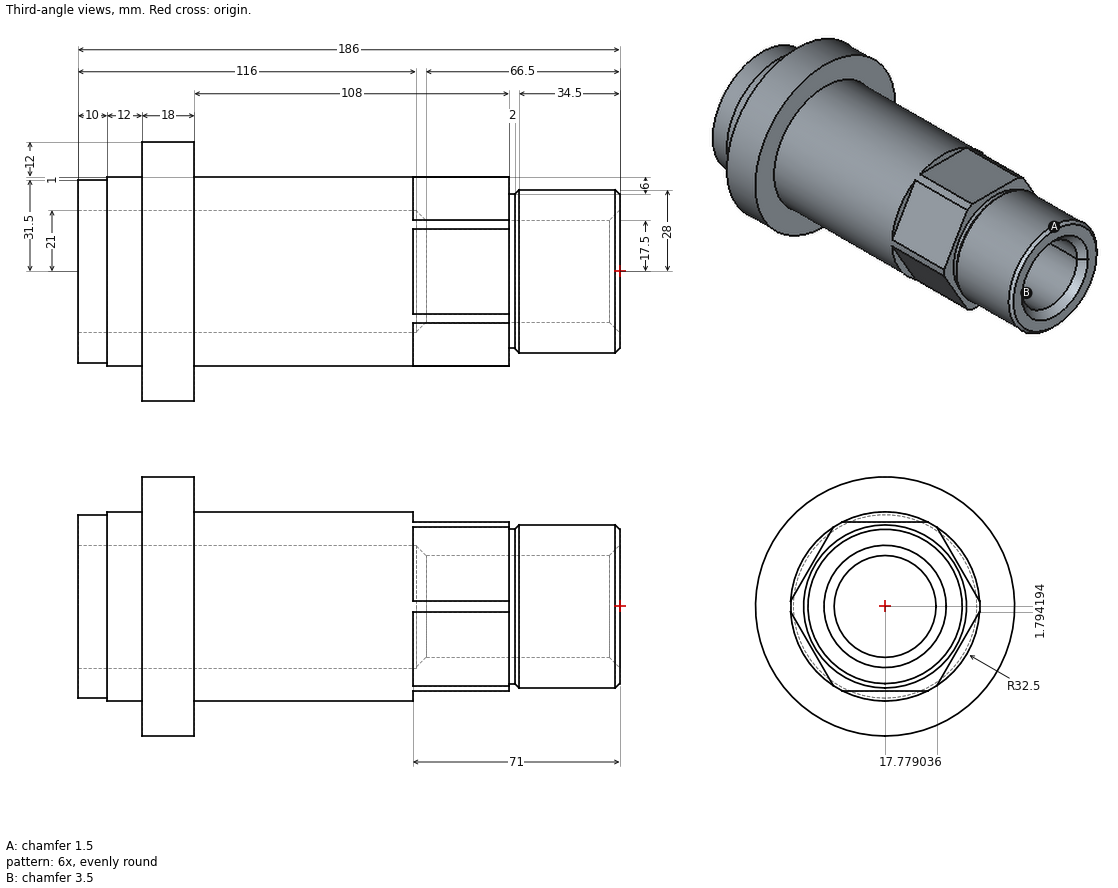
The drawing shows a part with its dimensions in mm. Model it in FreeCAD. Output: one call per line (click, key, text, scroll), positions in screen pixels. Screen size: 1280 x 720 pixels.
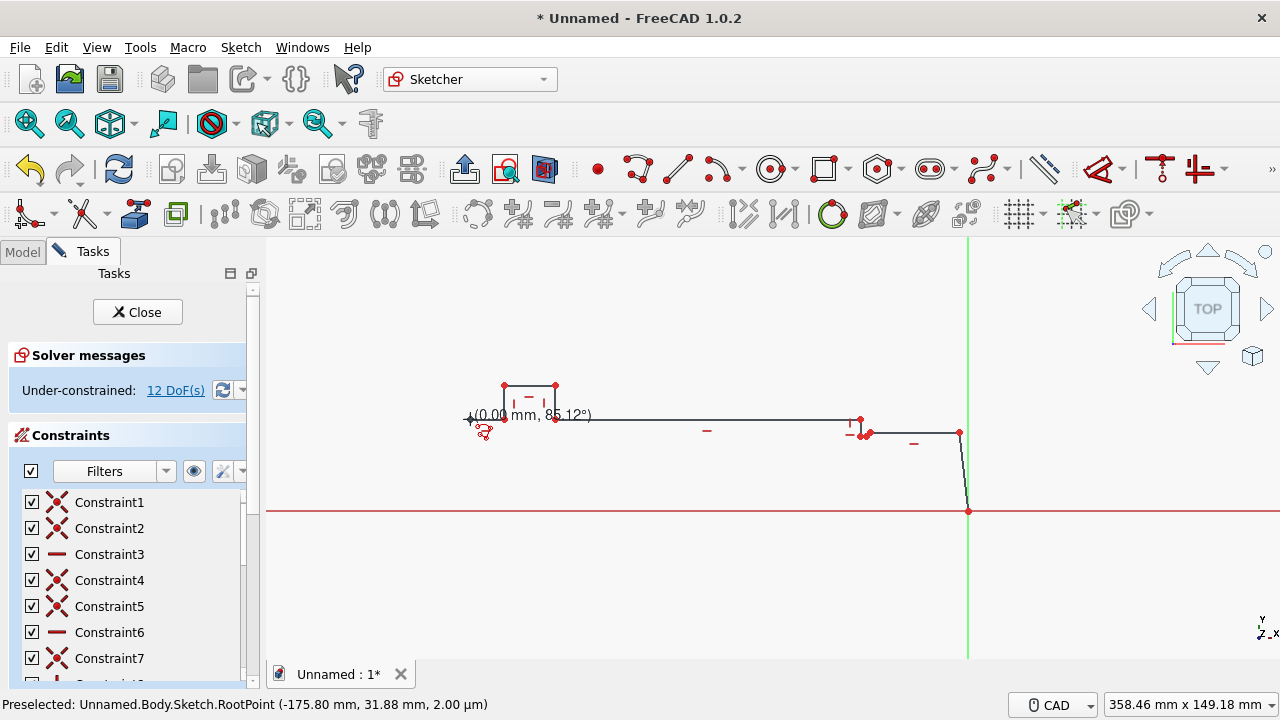
scroll(470, 422, up, 9)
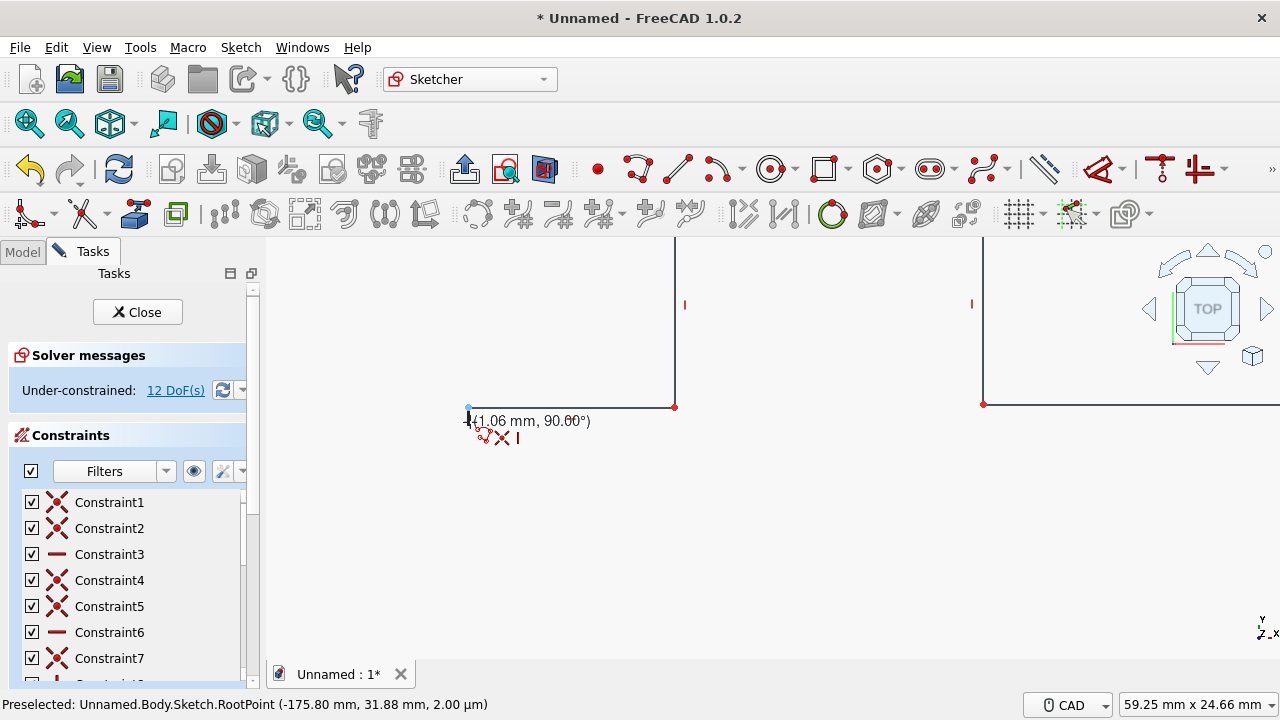
click(469, 420)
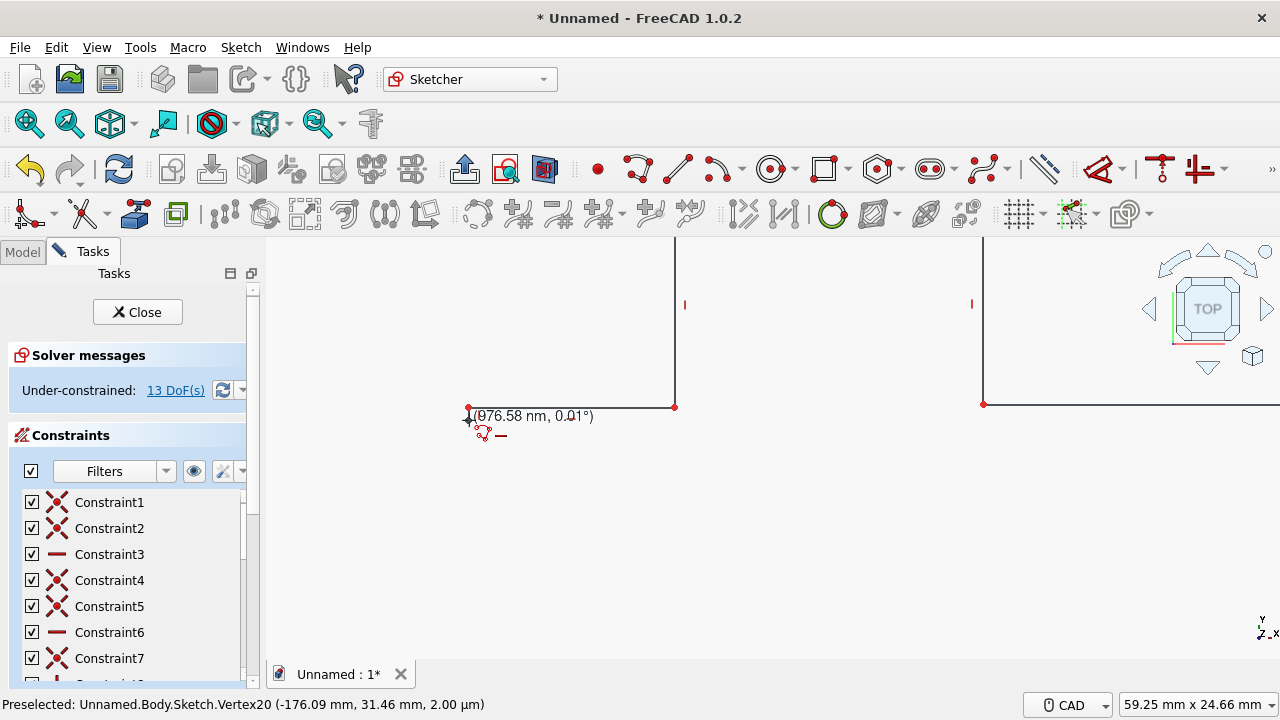
scroll(469, 422, down, 9)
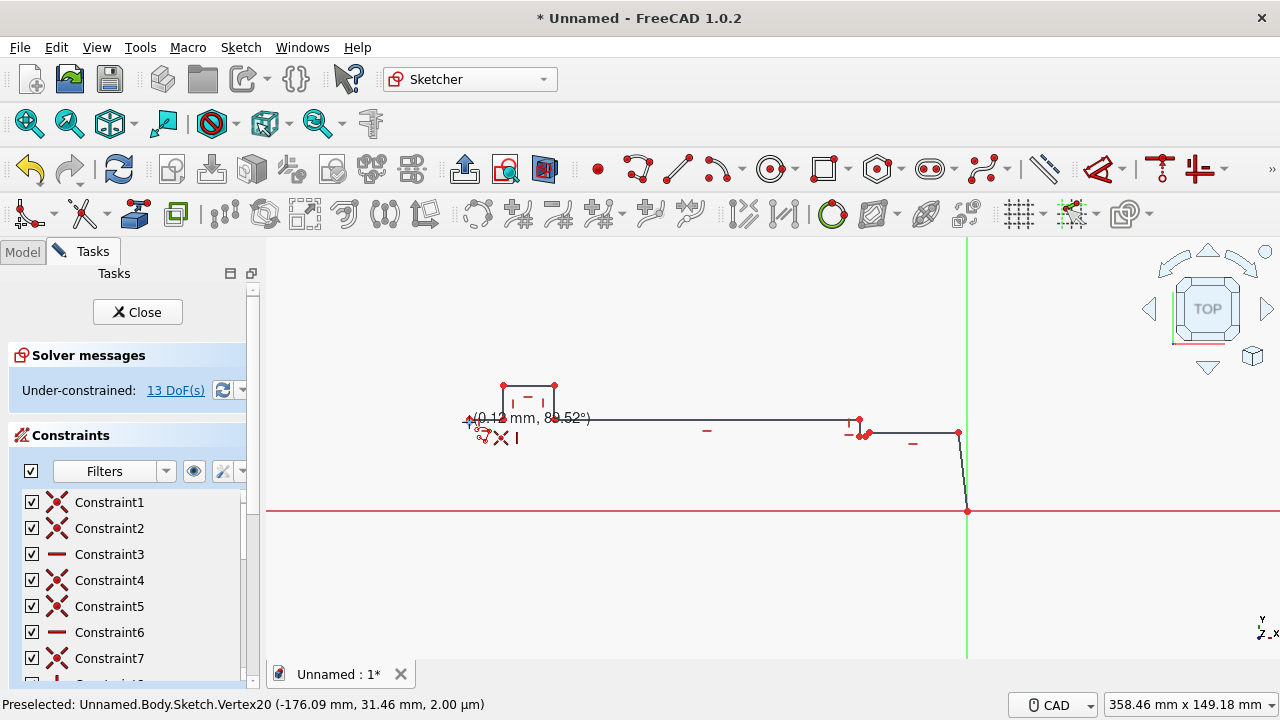
click(441, 422)
click(441, 502)
click(967, 511)
key(Escape)
key(Escape)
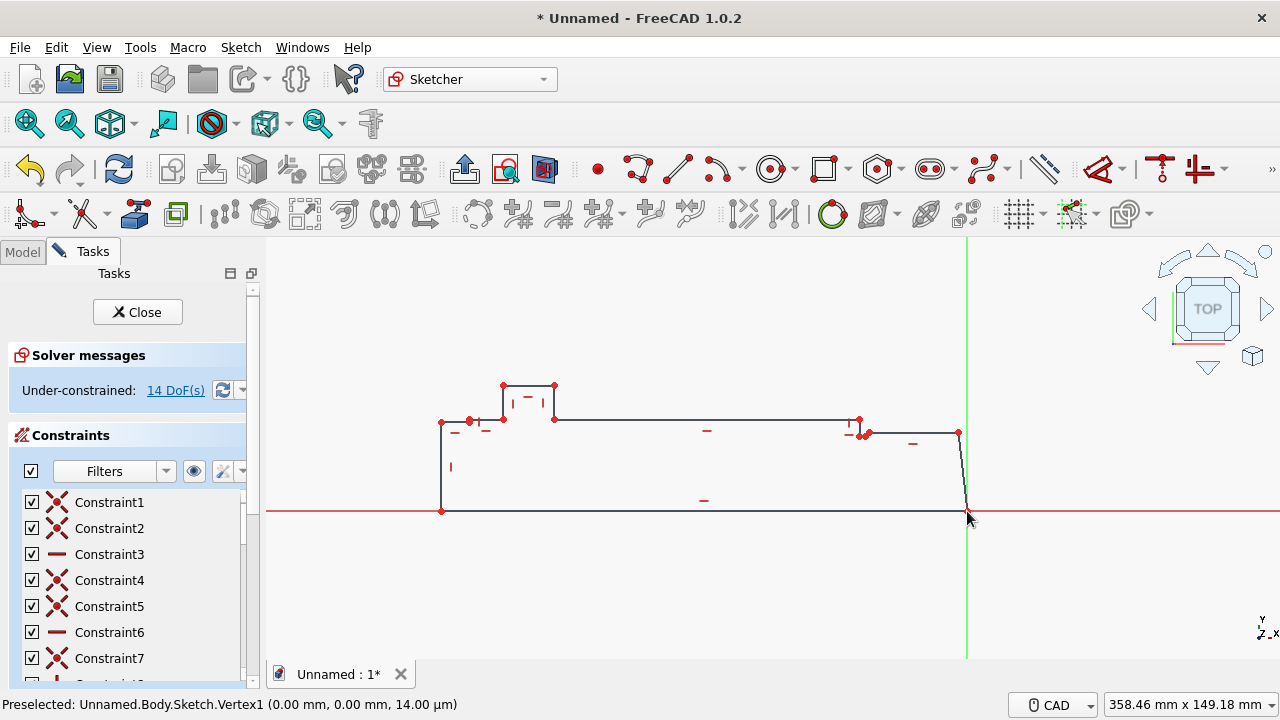
click(965, 488)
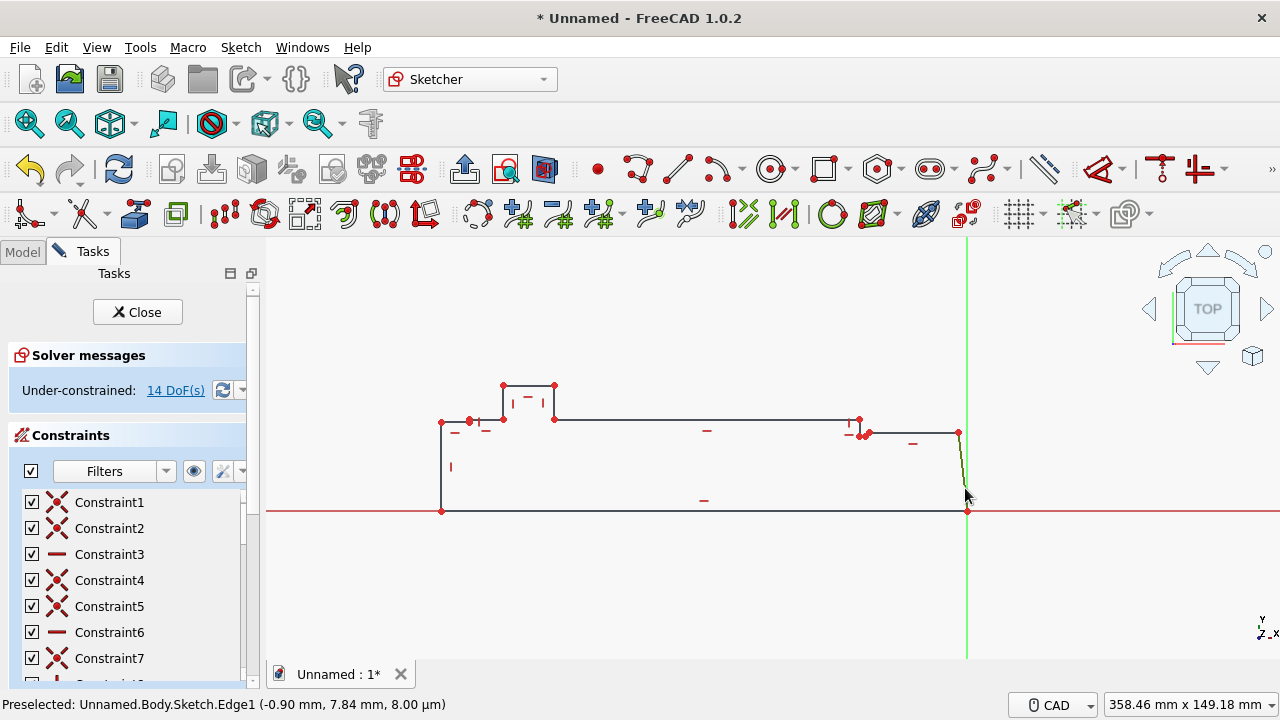
click(1226, 170)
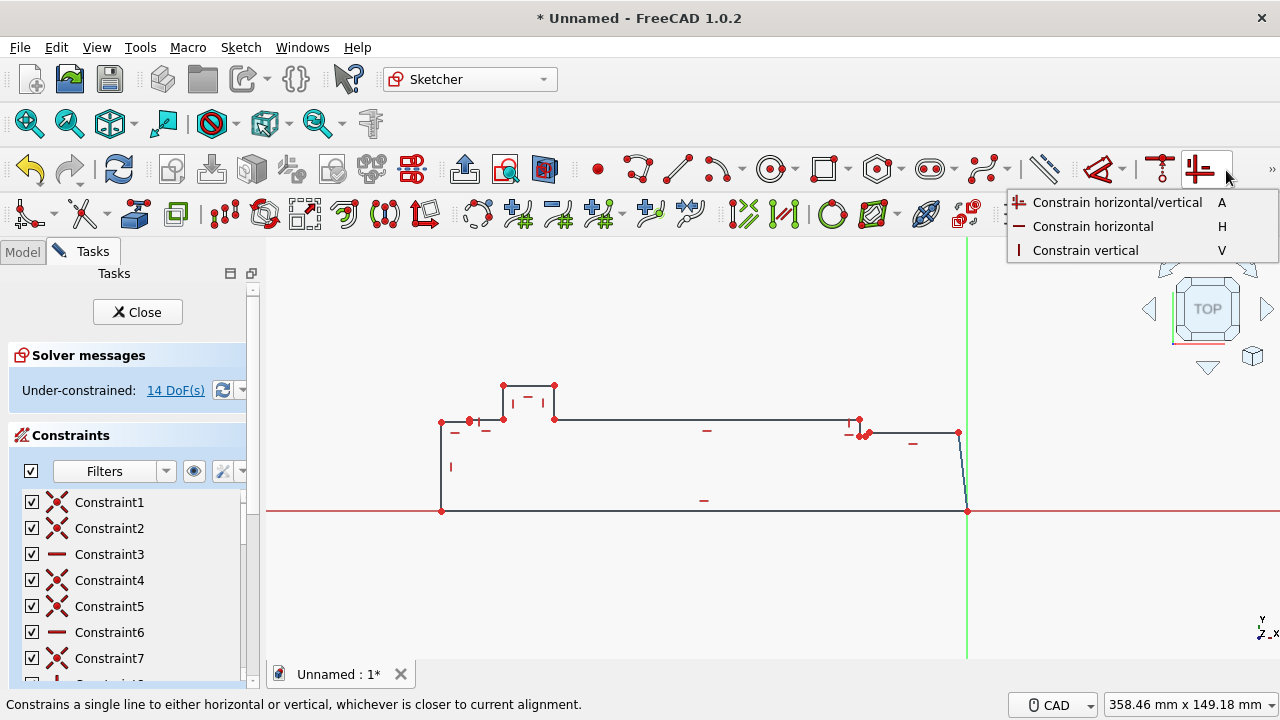
click(1143, 250)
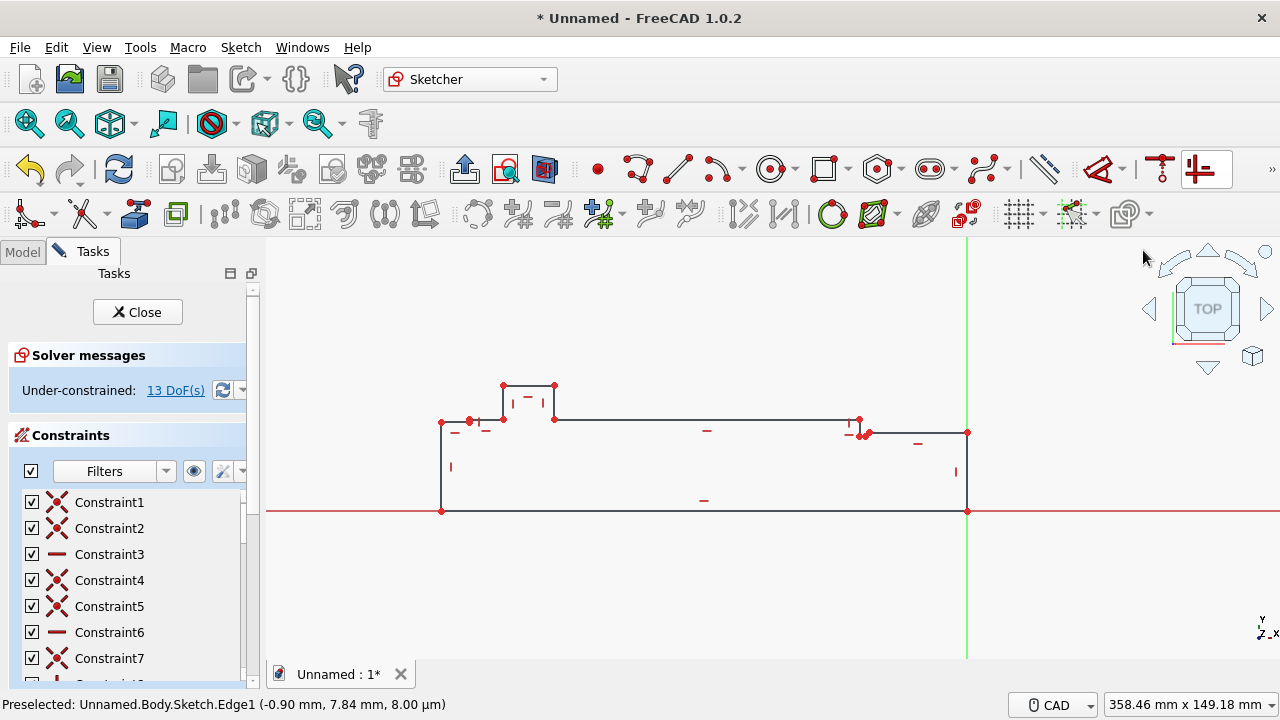
click(1098, 170)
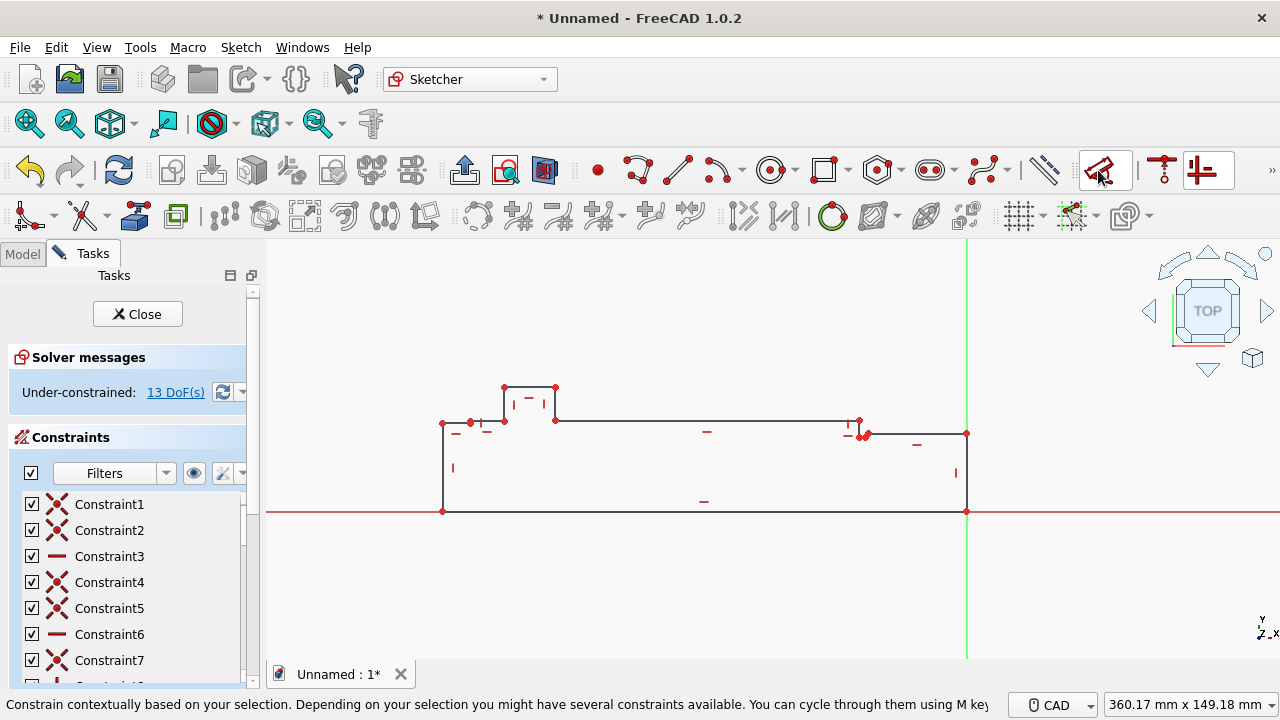
scroll(862, 438, up, 10)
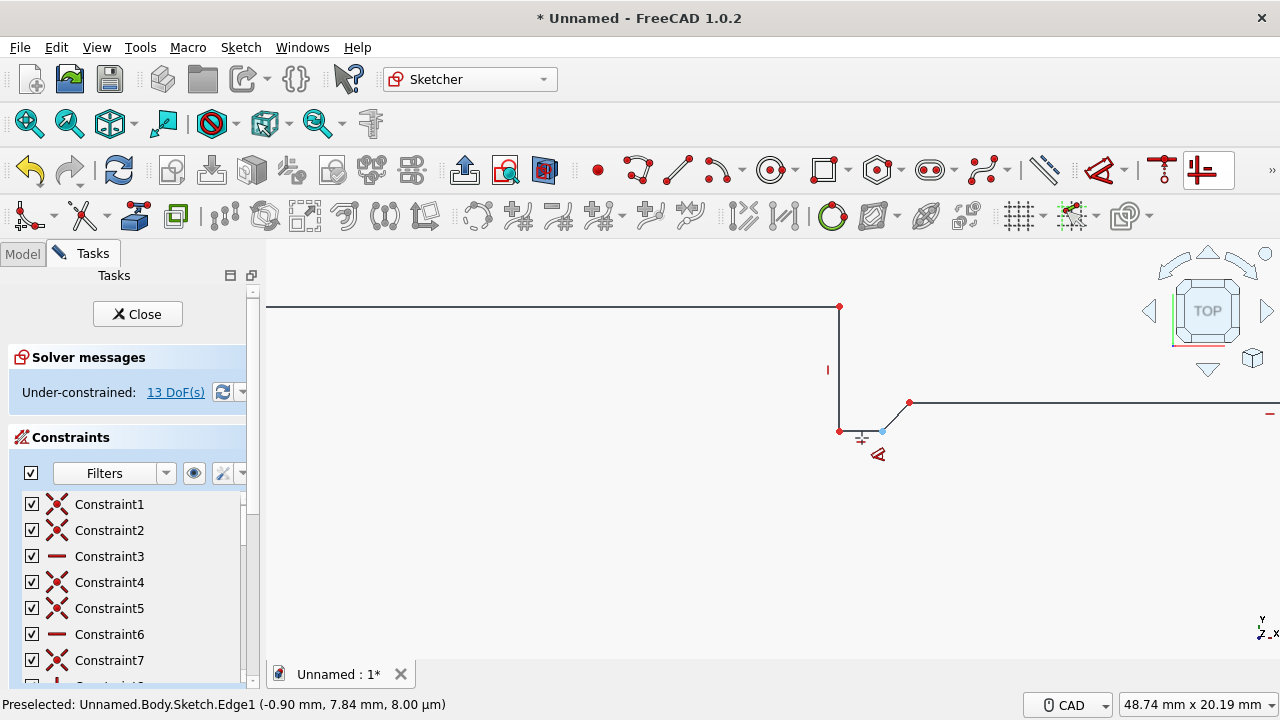
click(861, 431)
click(861, 397)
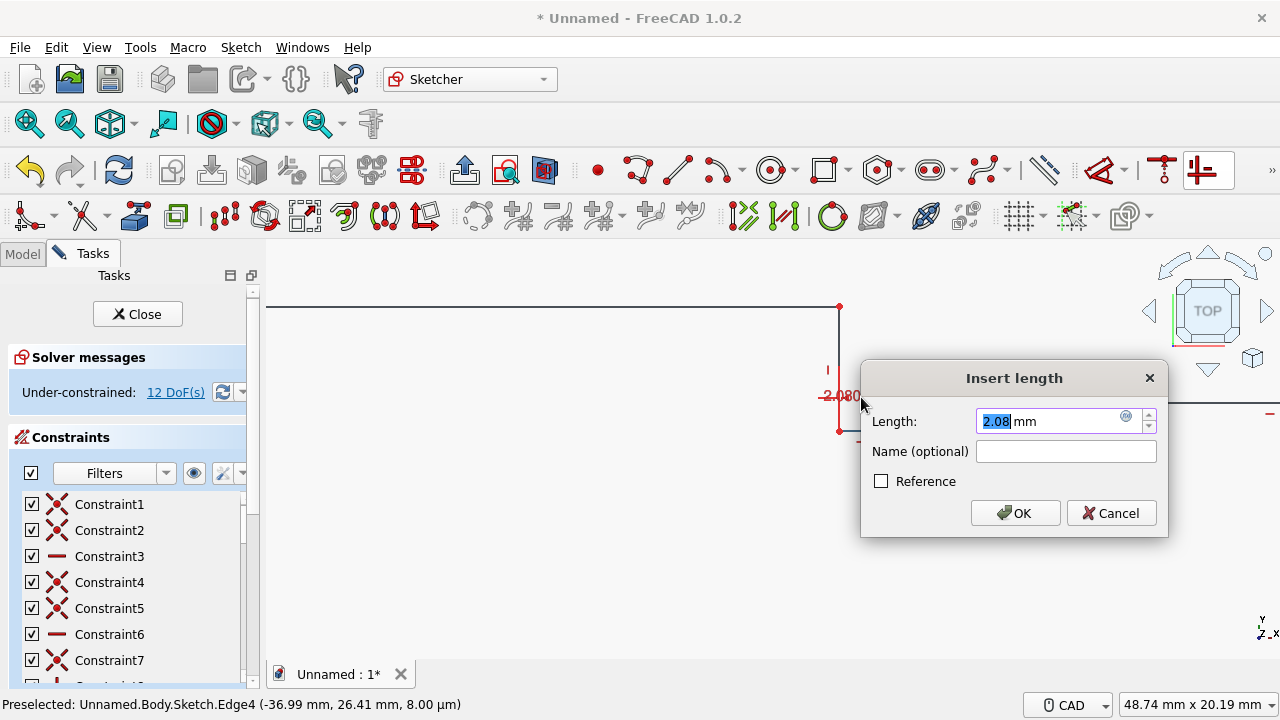
text(2)
key(Return)